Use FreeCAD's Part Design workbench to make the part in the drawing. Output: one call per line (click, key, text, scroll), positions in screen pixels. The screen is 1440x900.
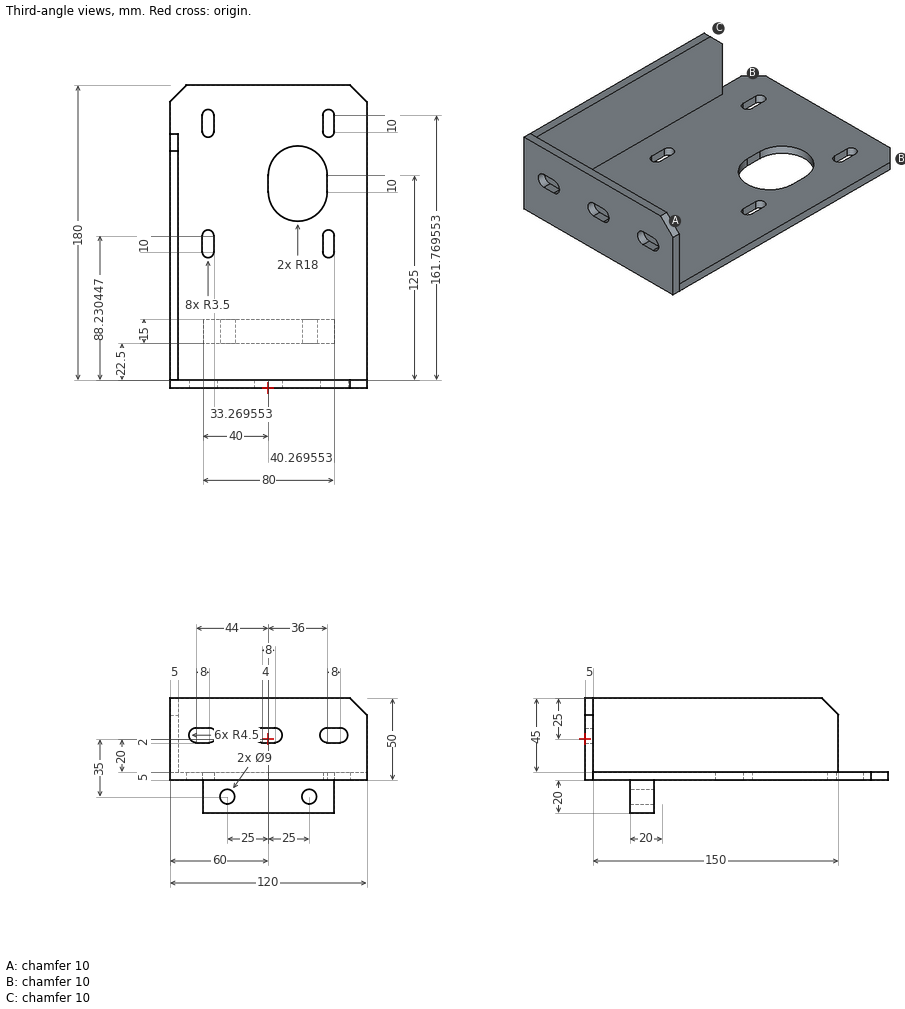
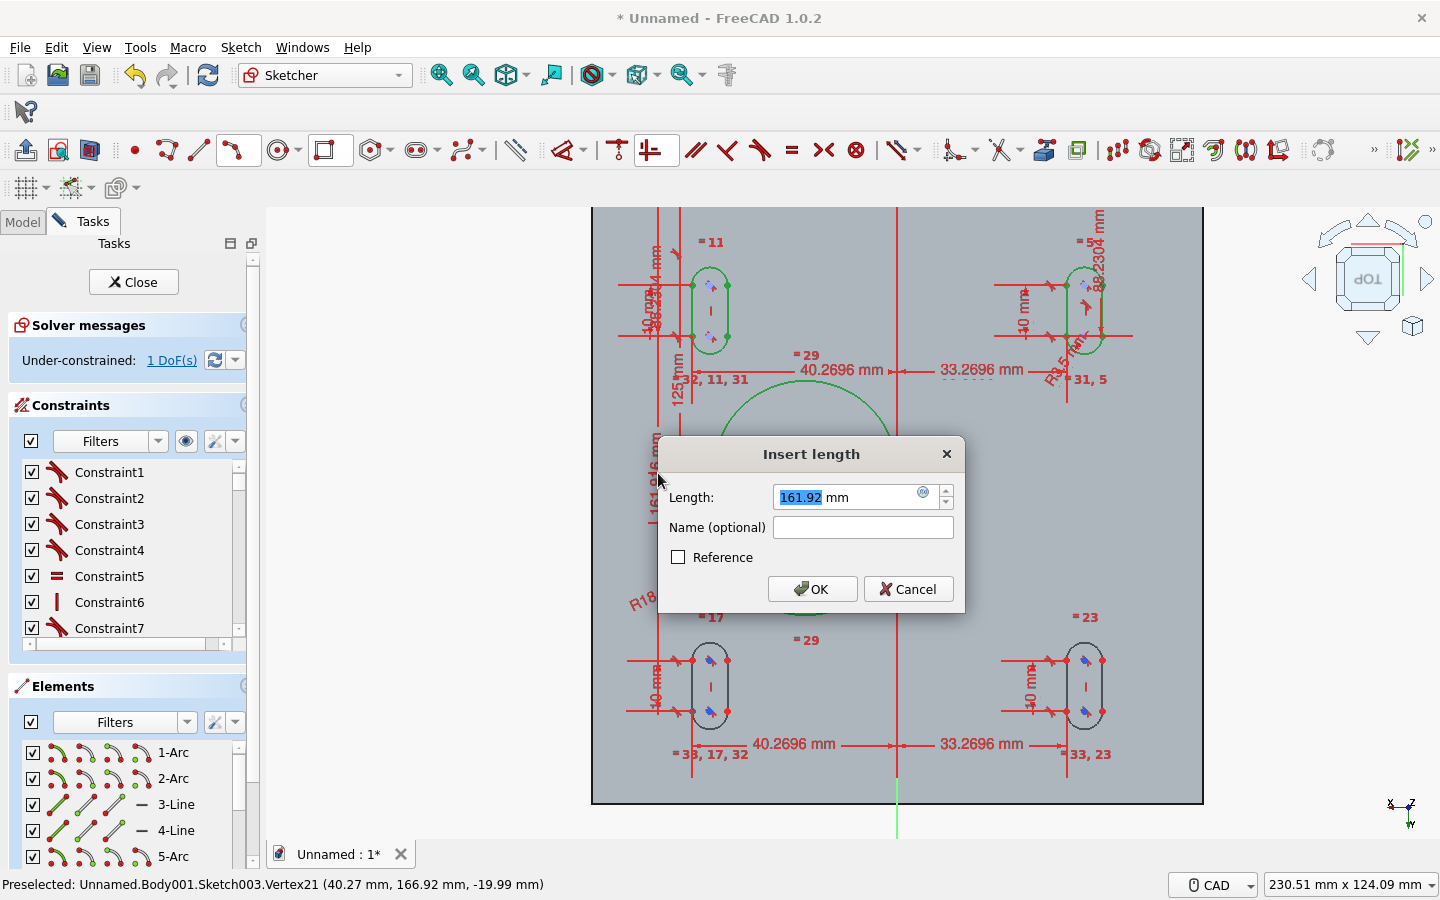
text(161.769553)
key(Return)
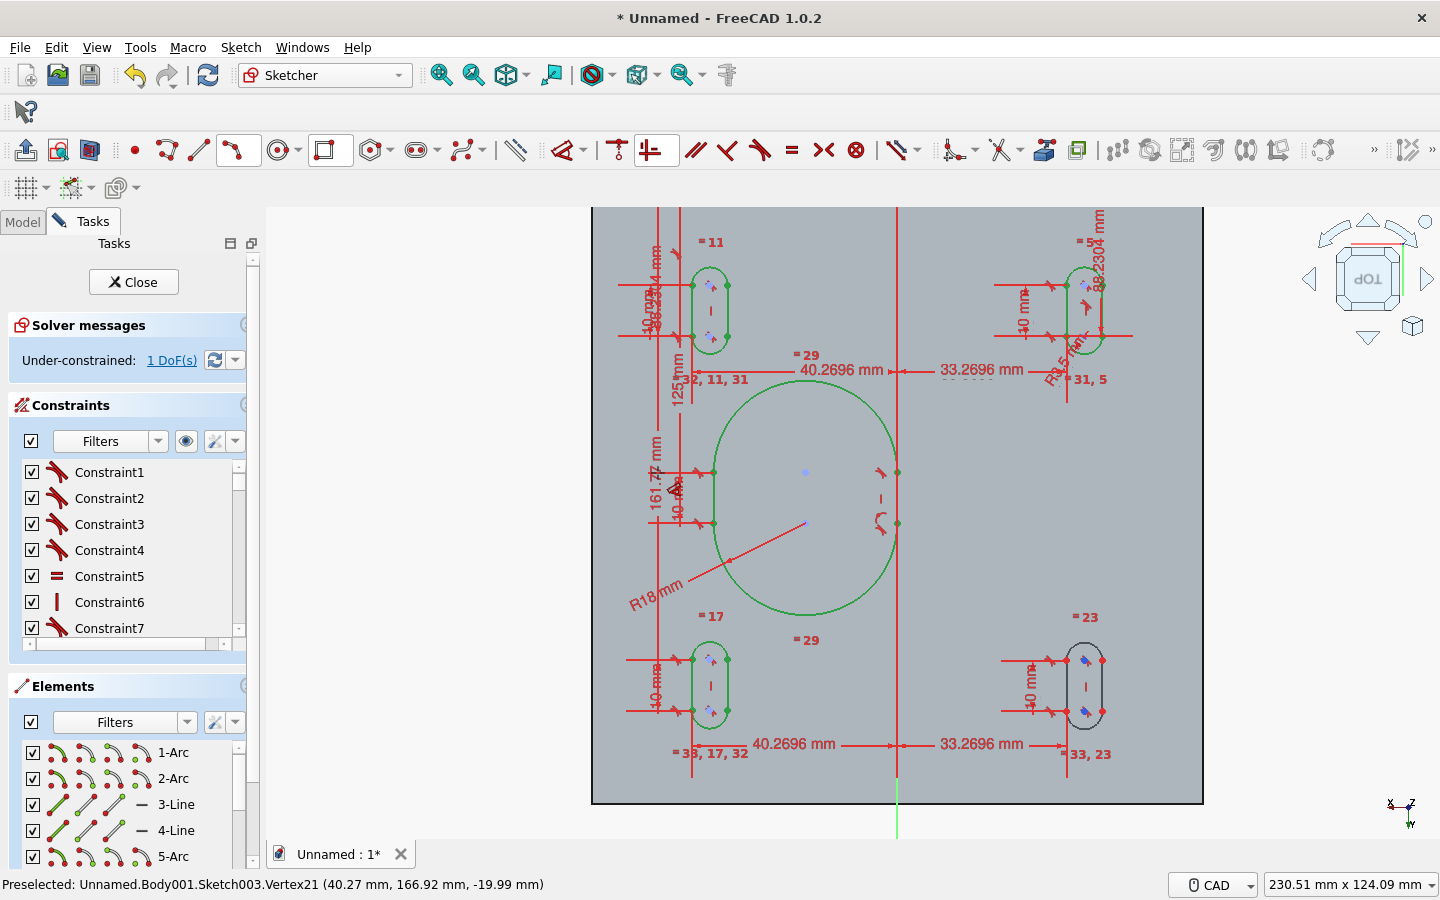
click(1067, 711)
click(1101, 473)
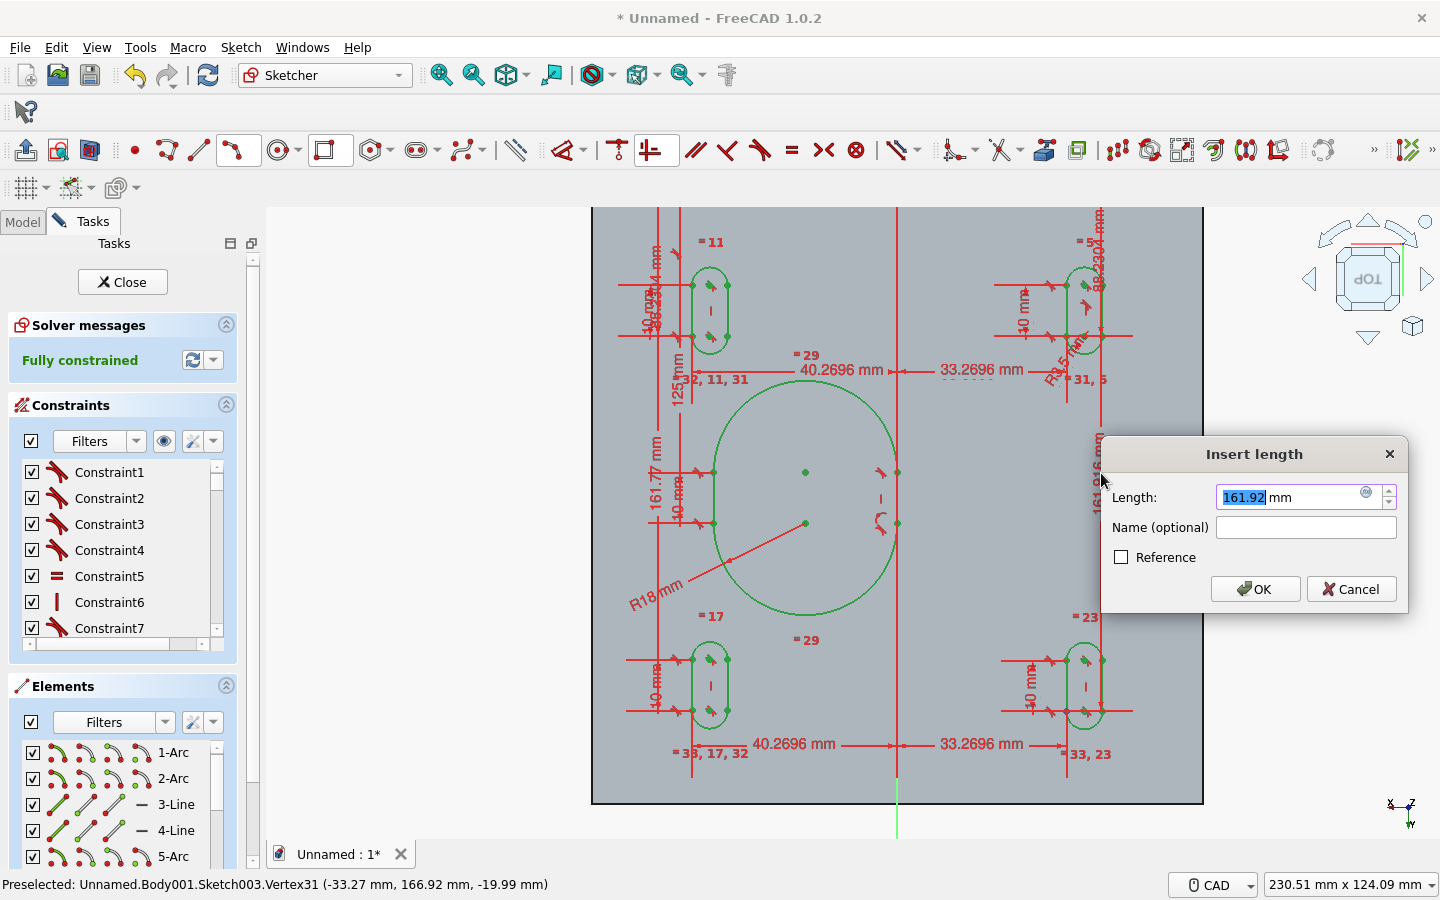
text(161.769553)
key(Return)
key(Escape)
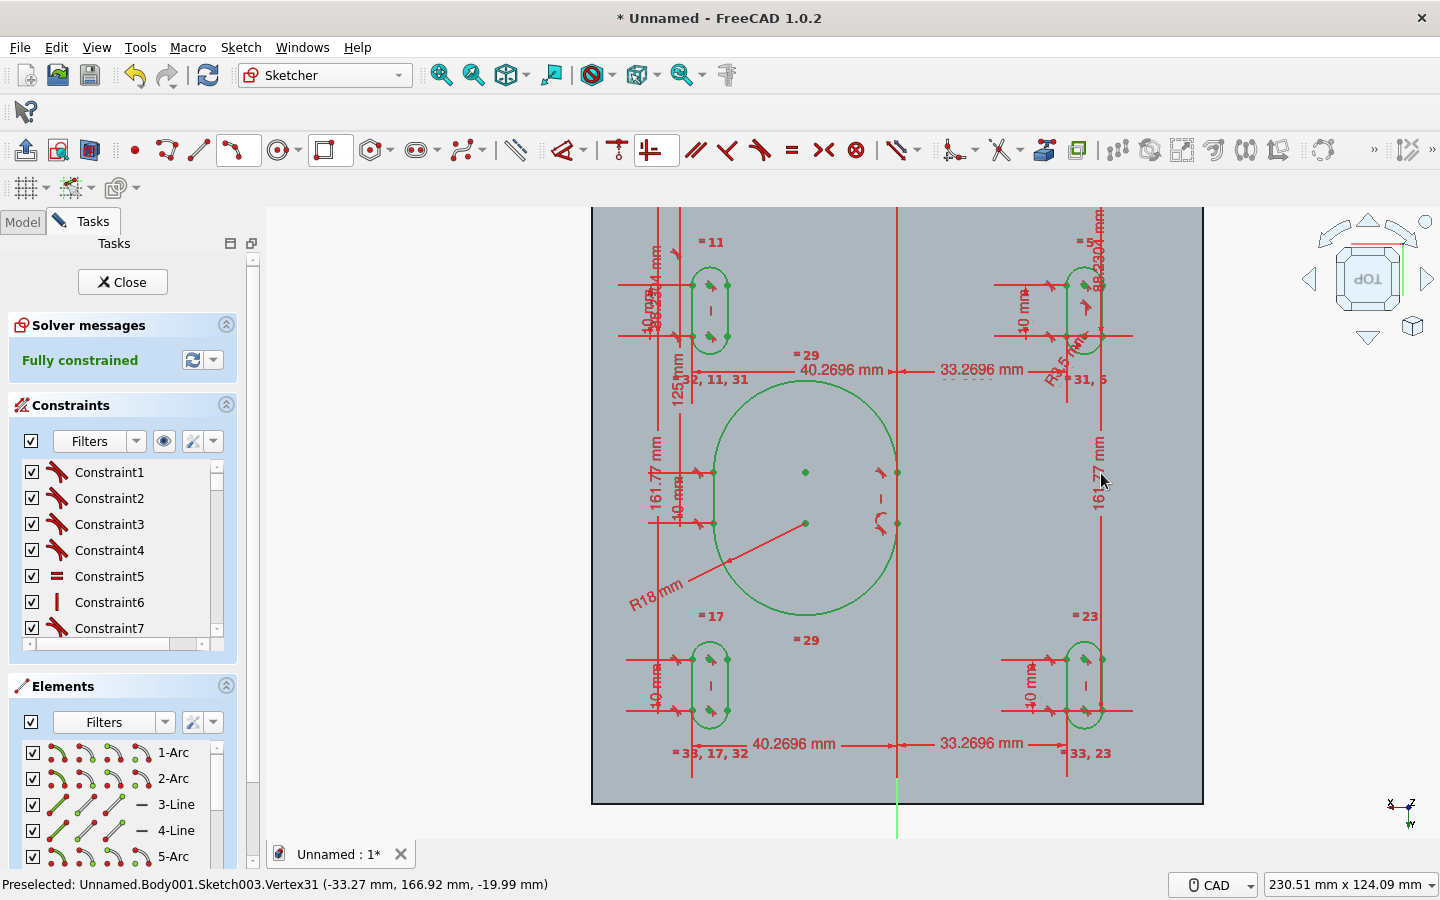
click(123, 282)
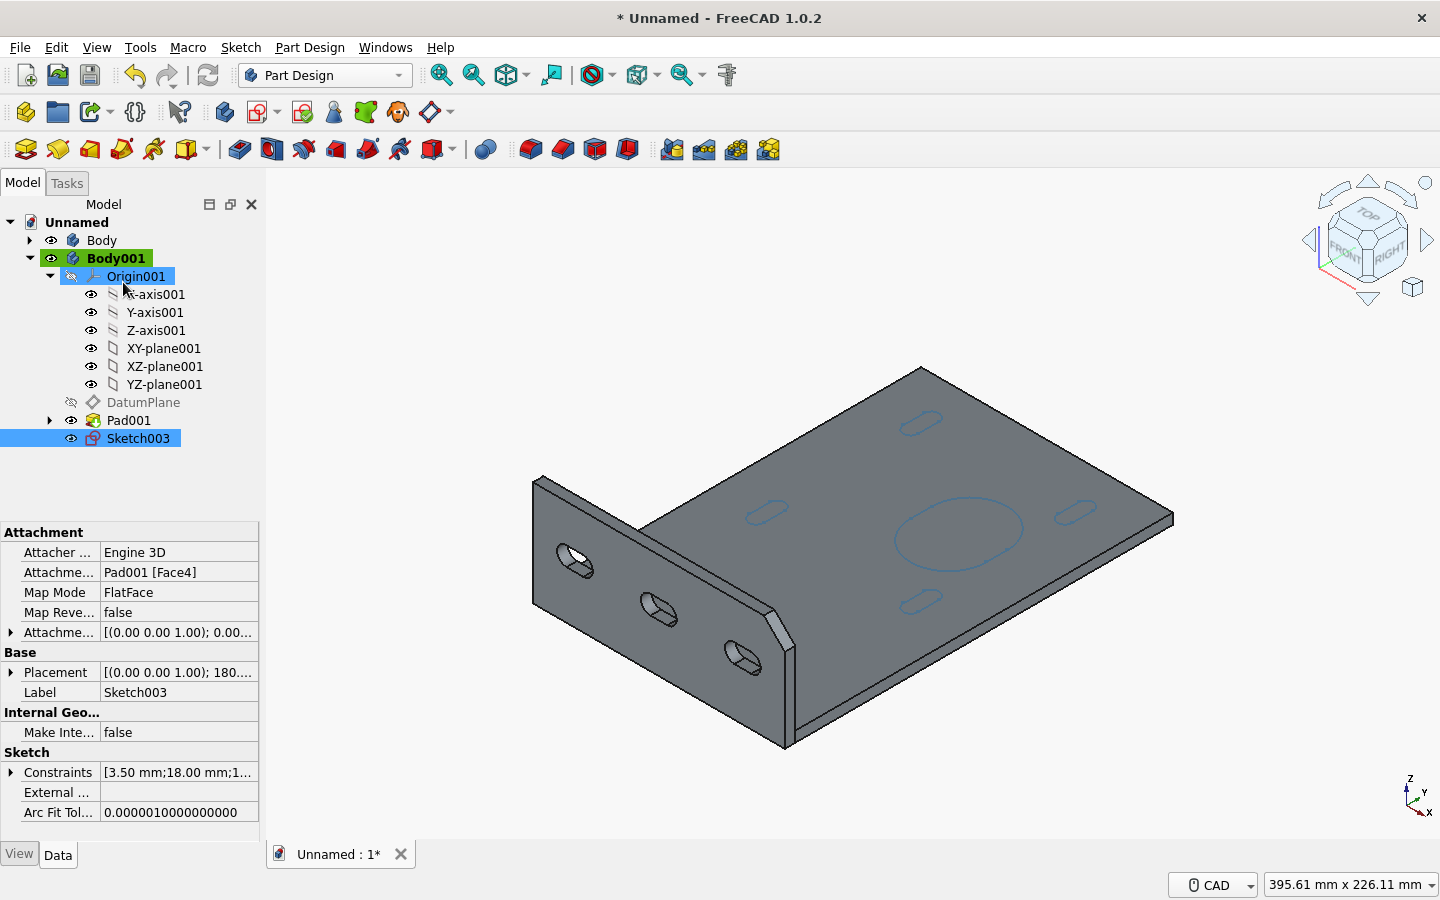
click(240, 150)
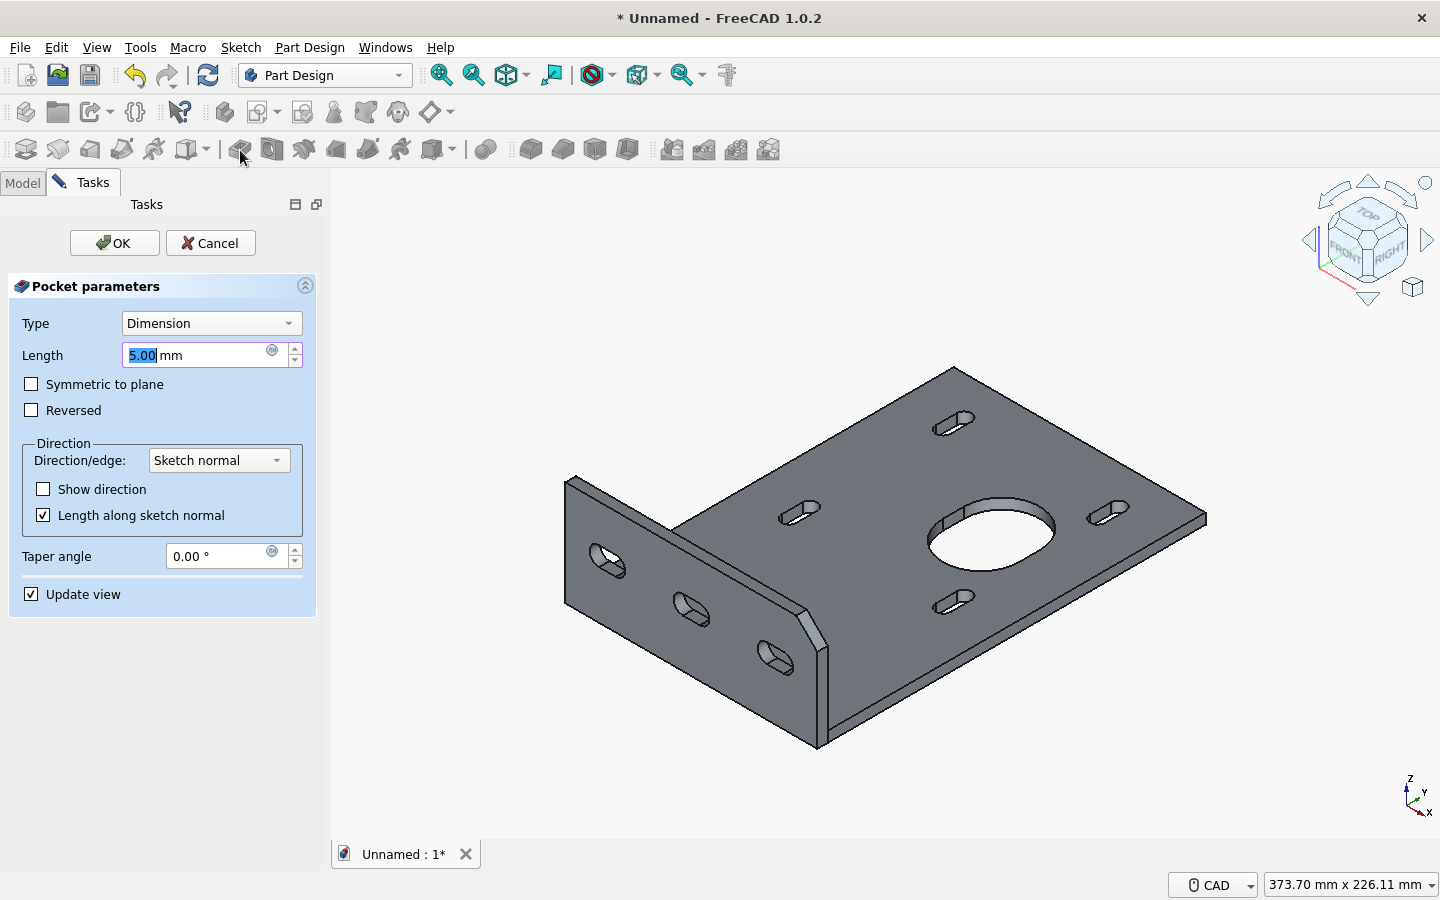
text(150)
key(Tab)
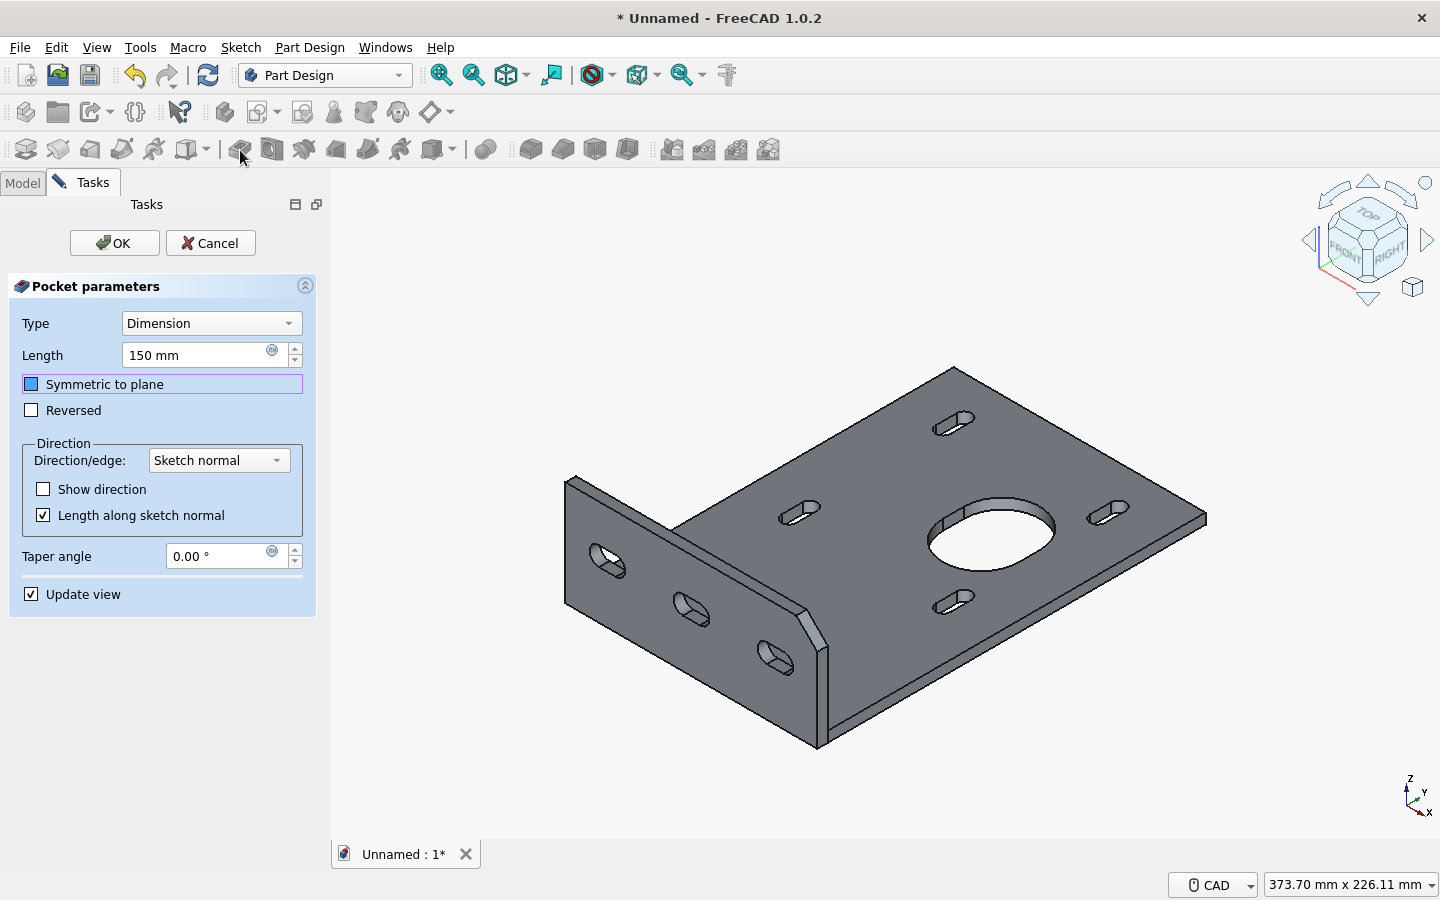
click(115, 243)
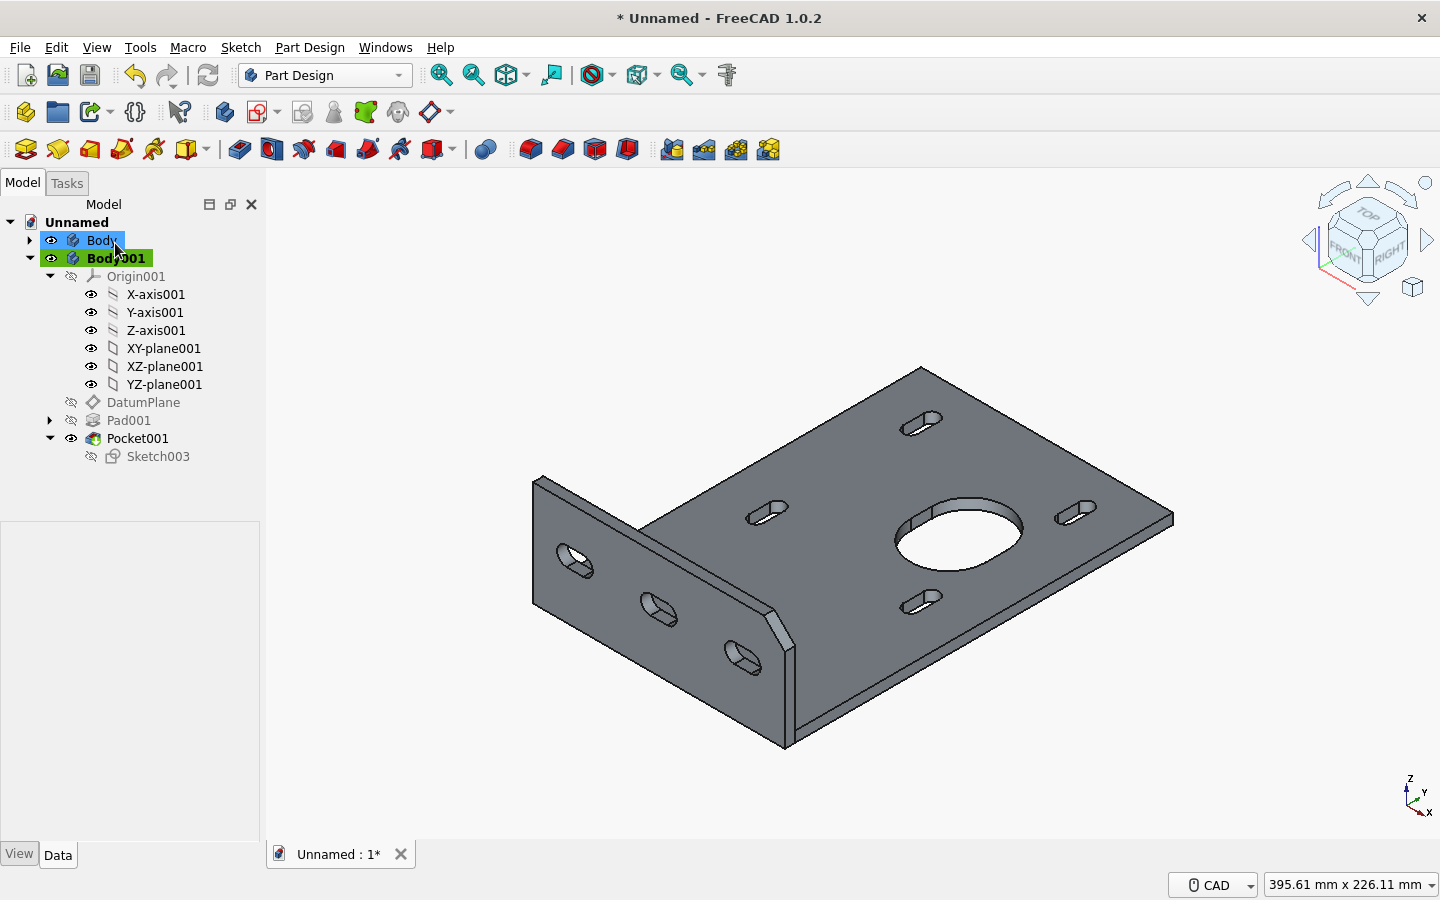
scroll(1173, 518, up, 5)